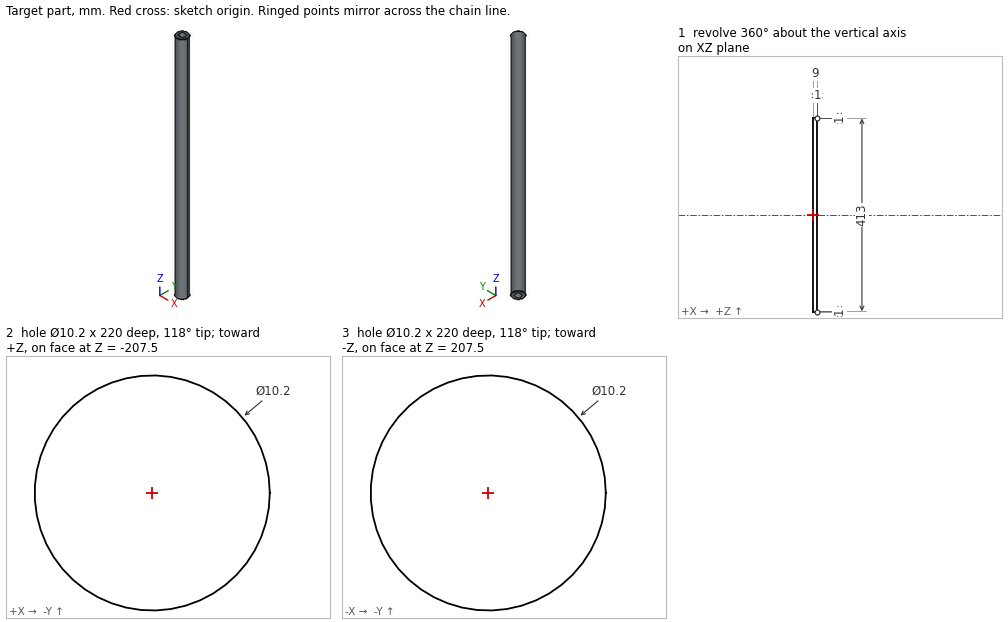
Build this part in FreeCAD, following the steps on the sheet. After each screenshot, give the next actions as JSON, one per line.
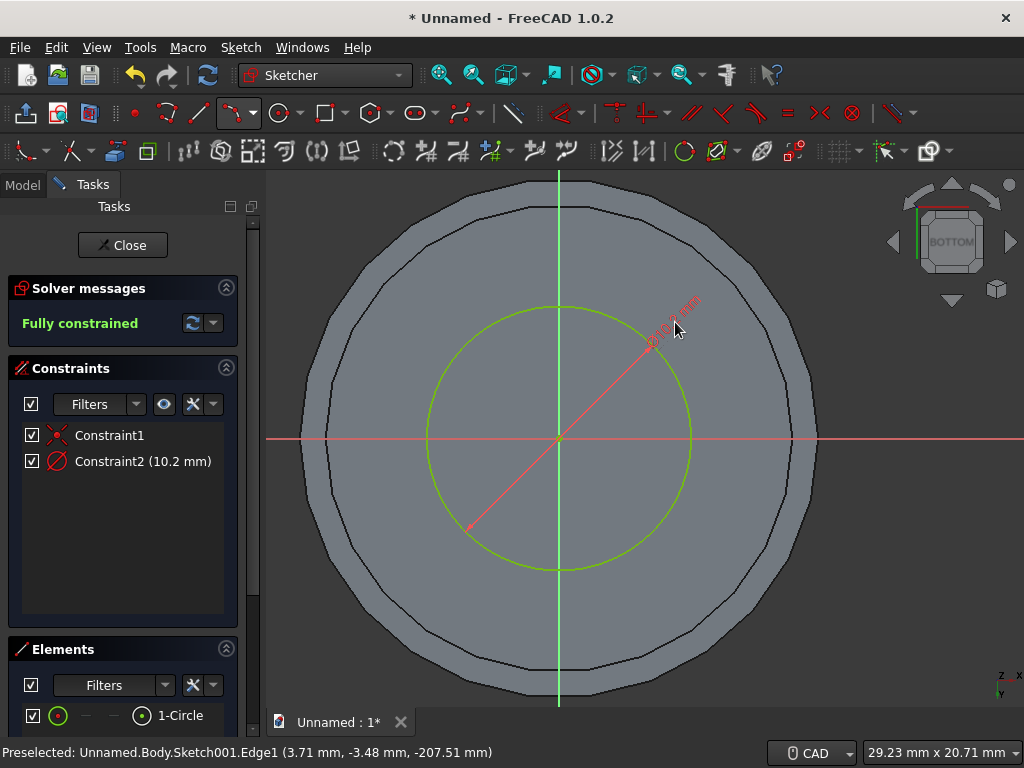
{"action": "left_click", "coordinate": [123, 245]}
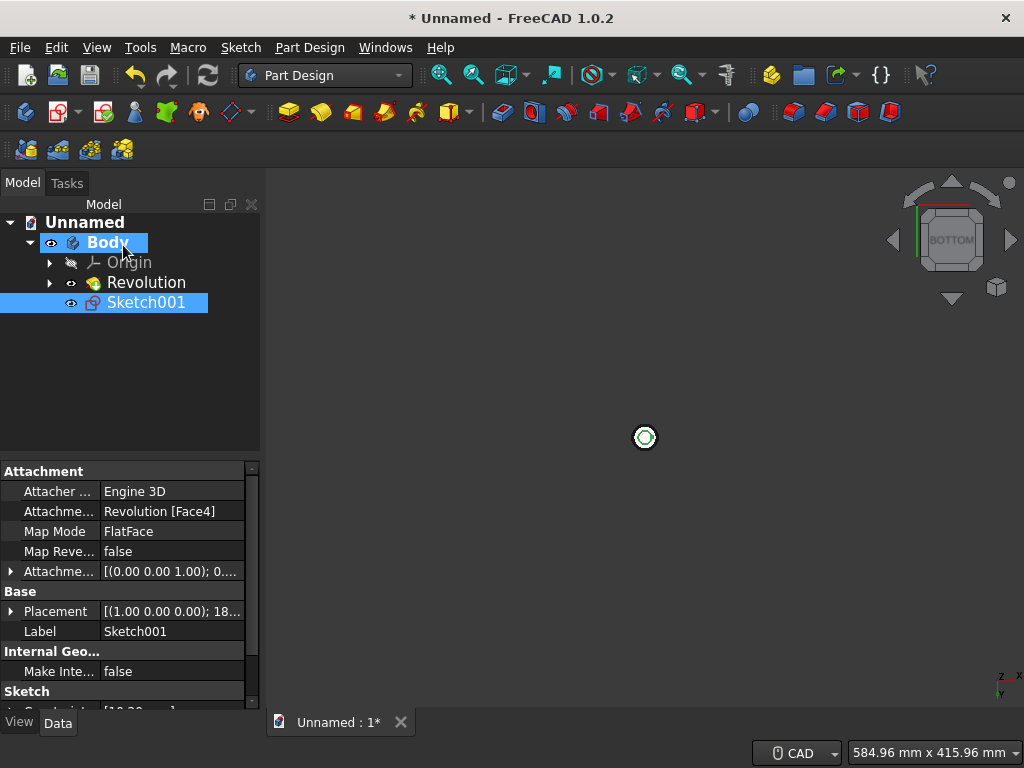
{"action": "left_click", "coordinate": [536, 112]}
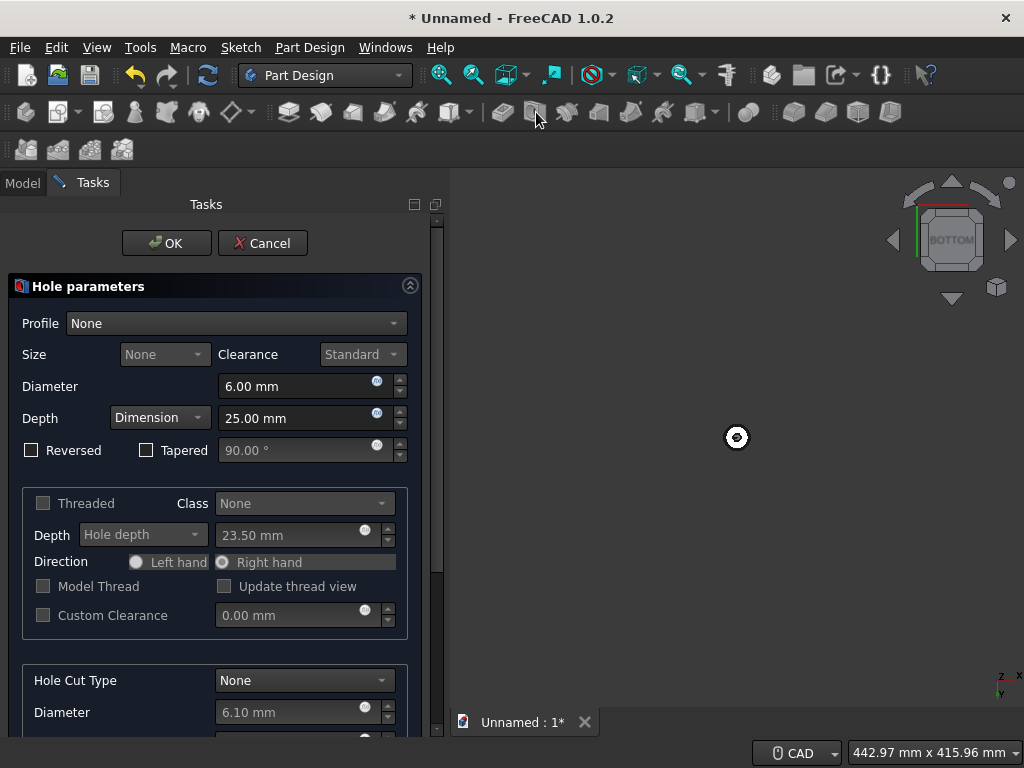
{"action": "triple_click", "coordinate": [305, 386]}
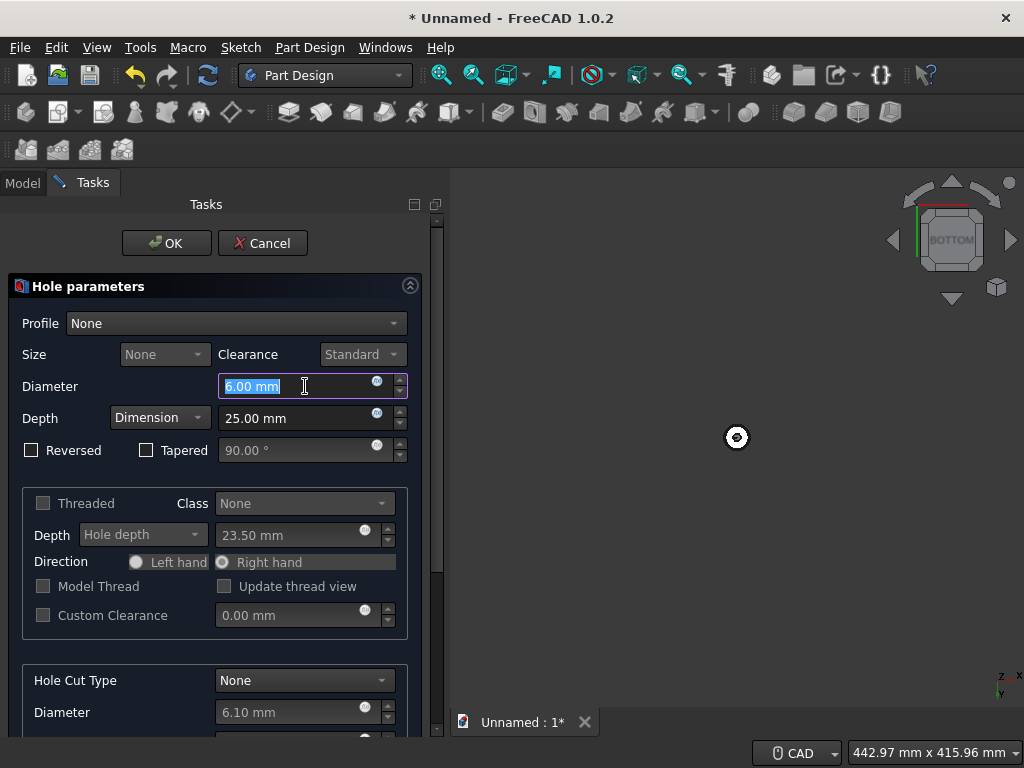
{"action": "type", "text": "10.2"}
{"action": "key", "text": "Tab"}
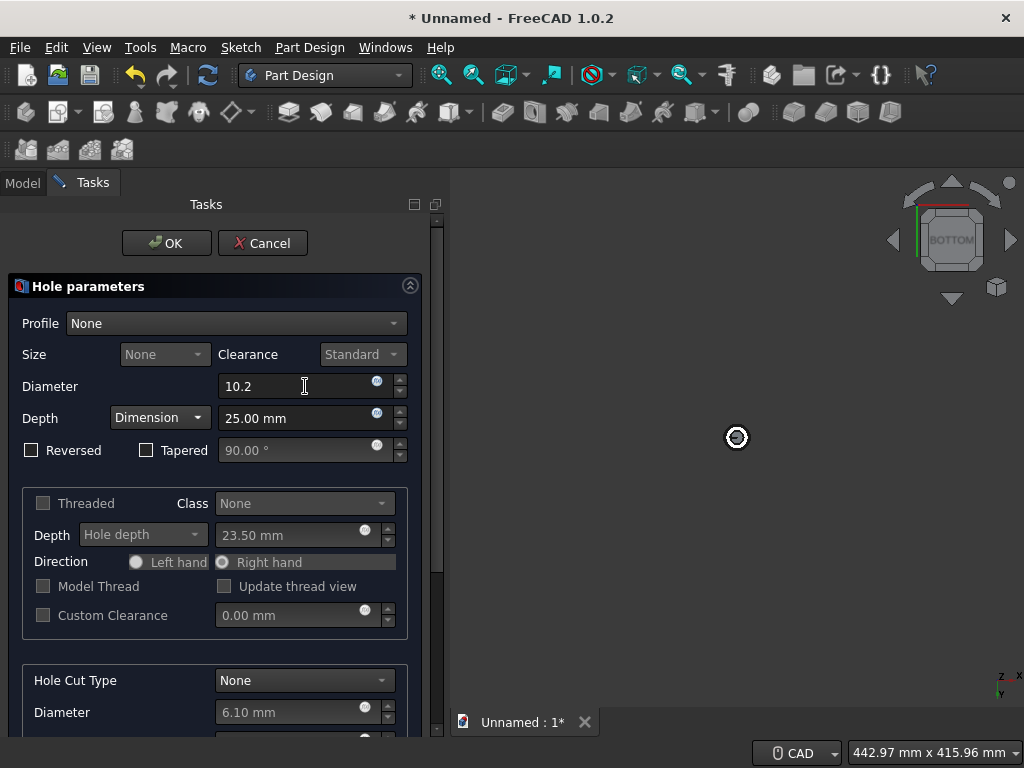
{"action": "triple_click", "coordinate": [305, 418]}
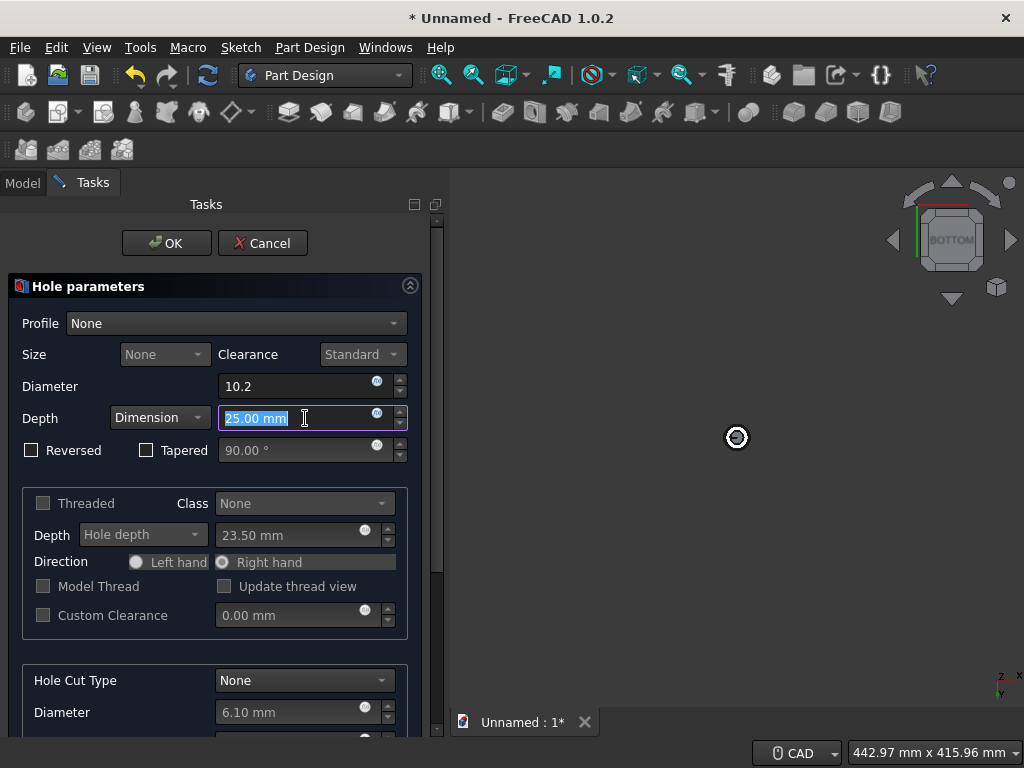
{"action": "type", "text": "220"}
{"action": "key", "text": "Tab"}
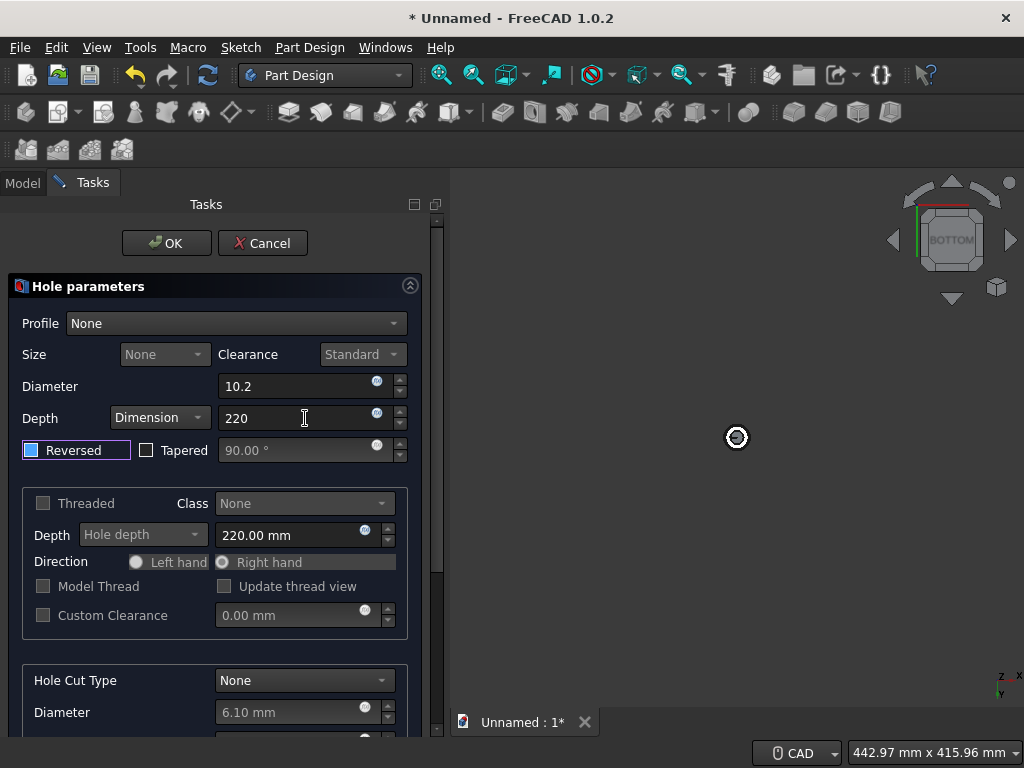
{"action": "left_click", "coordinate": [167, 243]}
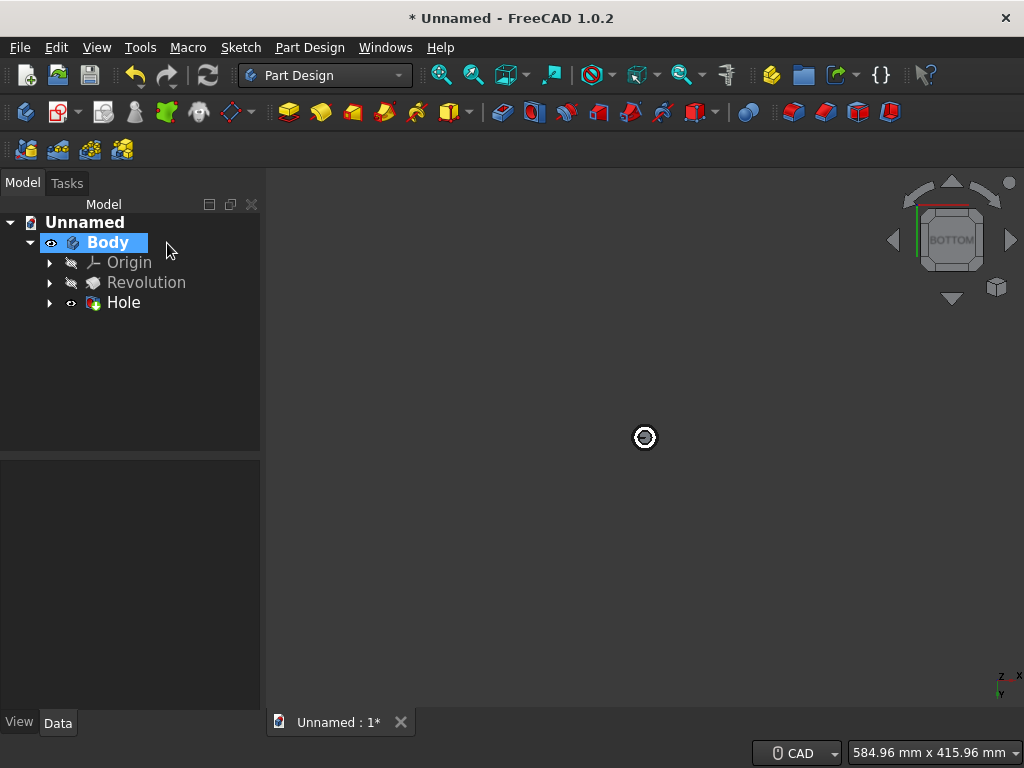
{"action": "key", "text": "v f"}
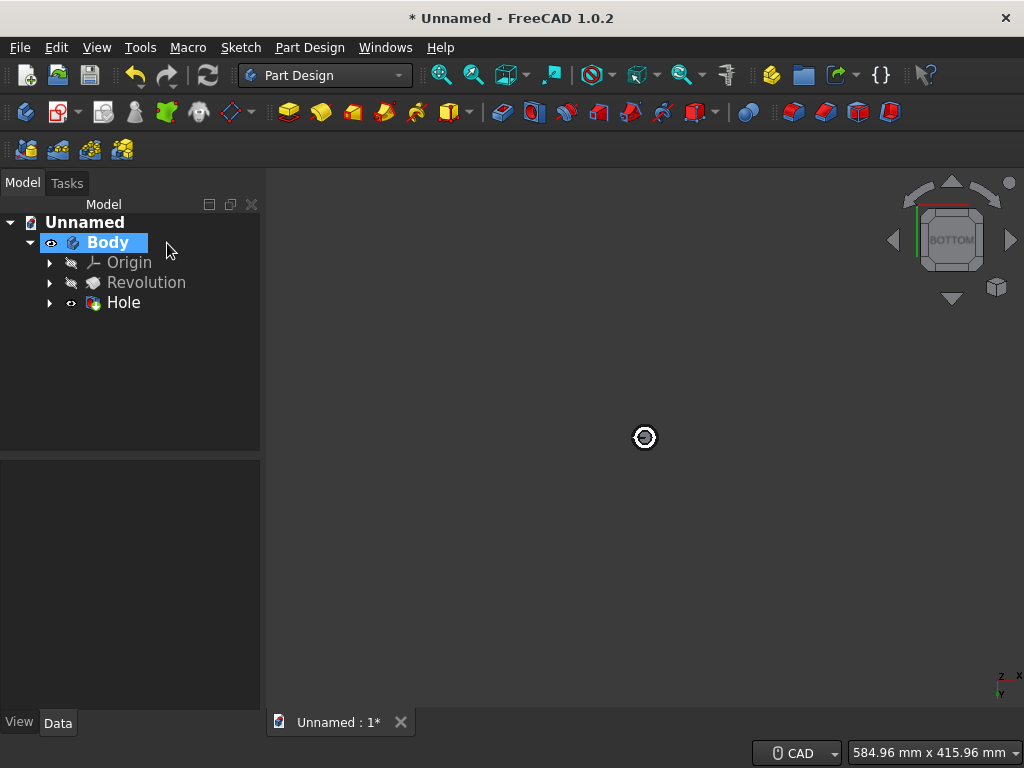
{"action": "key", "text": "0"}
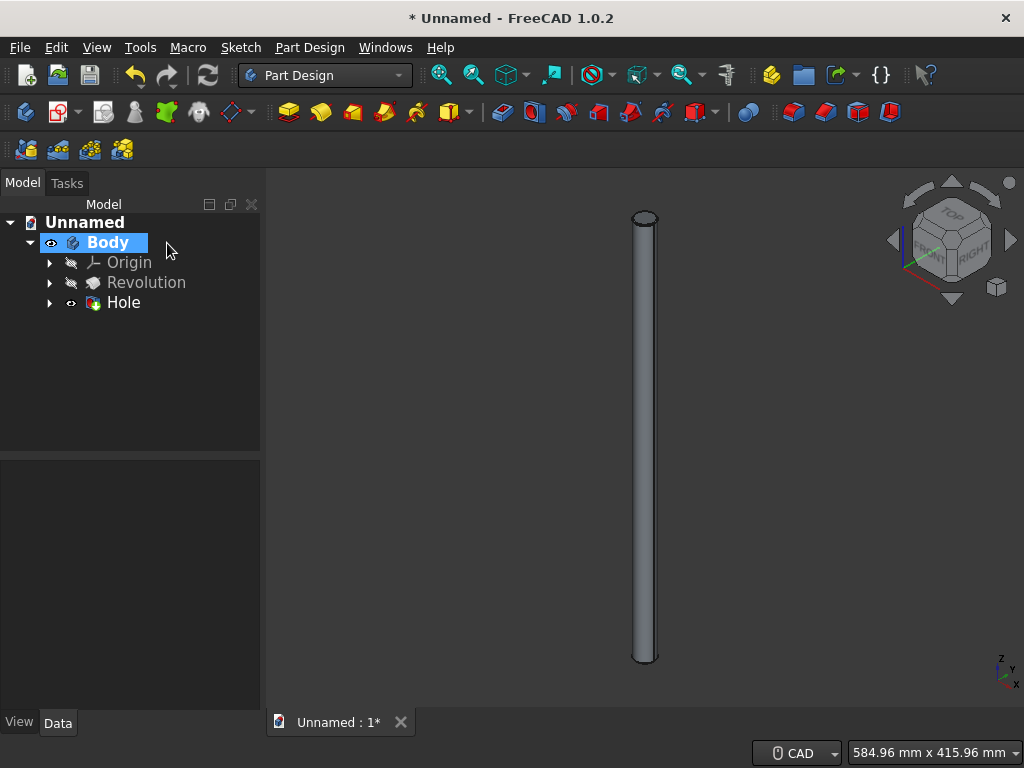
{"action": "key", "text": "2"}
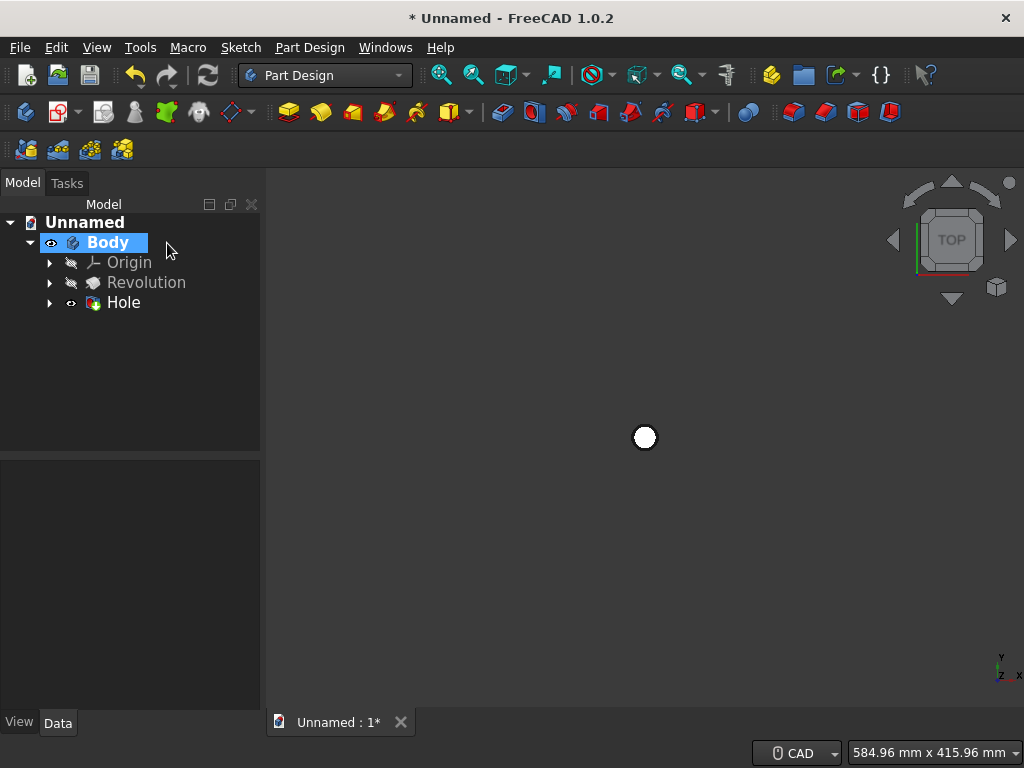
{"action": "key", "text": "v f"}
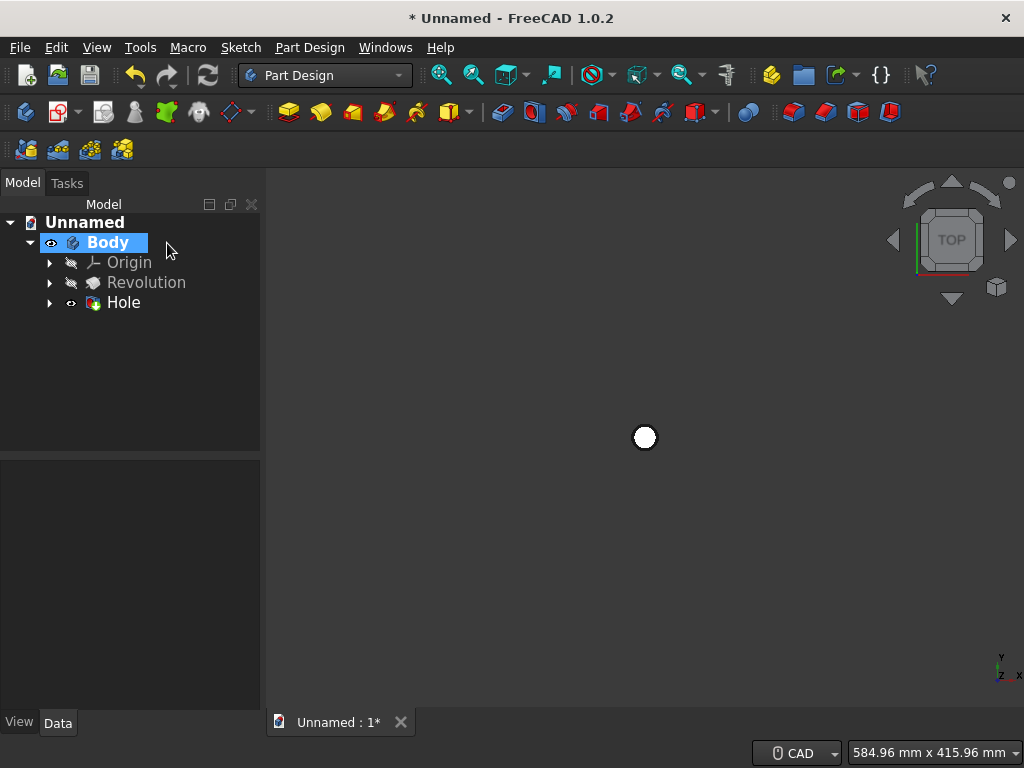
{"action": "left_click", "coordinate": [645, 436]}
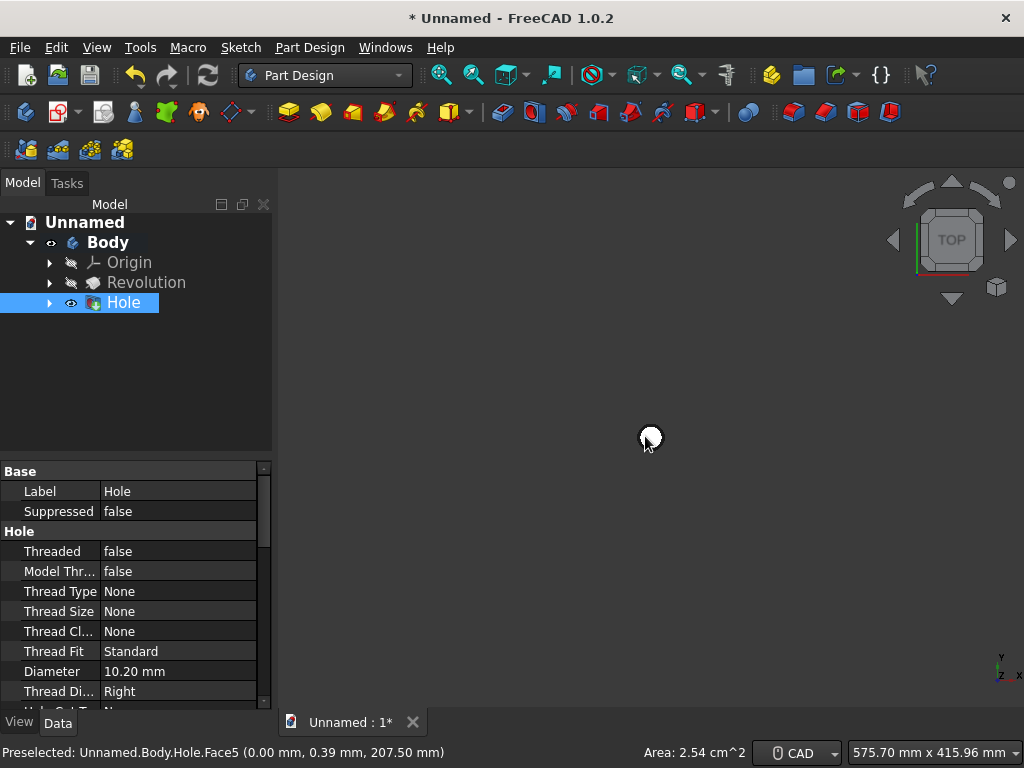
{"action": "left_click", "coordinate": [58, 112]}